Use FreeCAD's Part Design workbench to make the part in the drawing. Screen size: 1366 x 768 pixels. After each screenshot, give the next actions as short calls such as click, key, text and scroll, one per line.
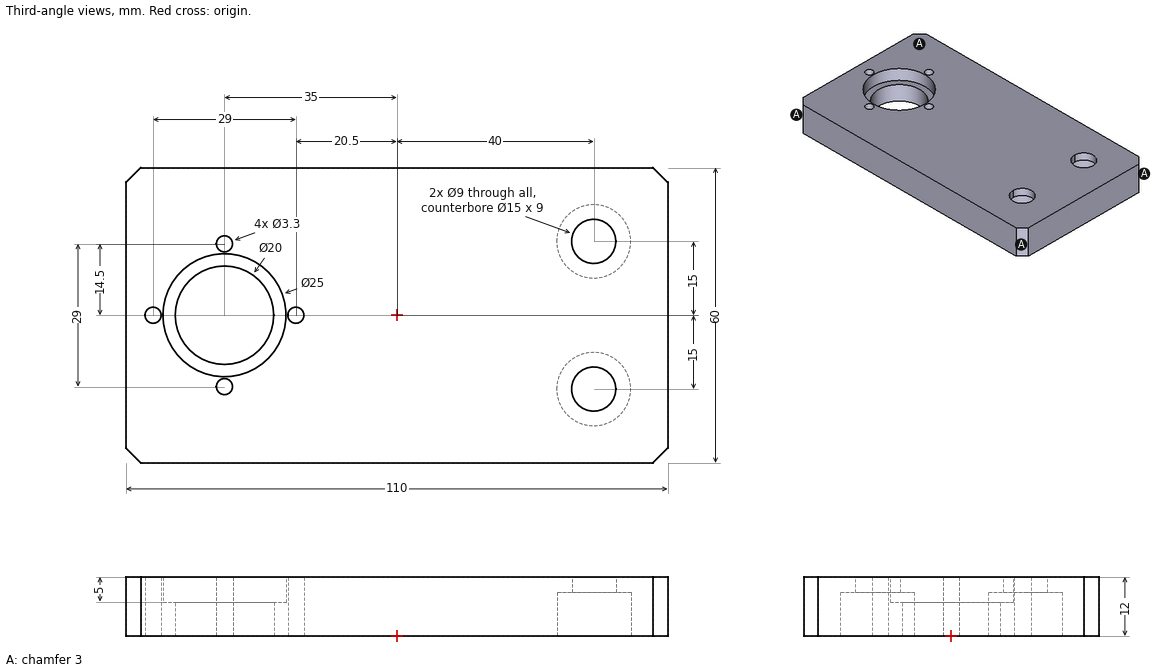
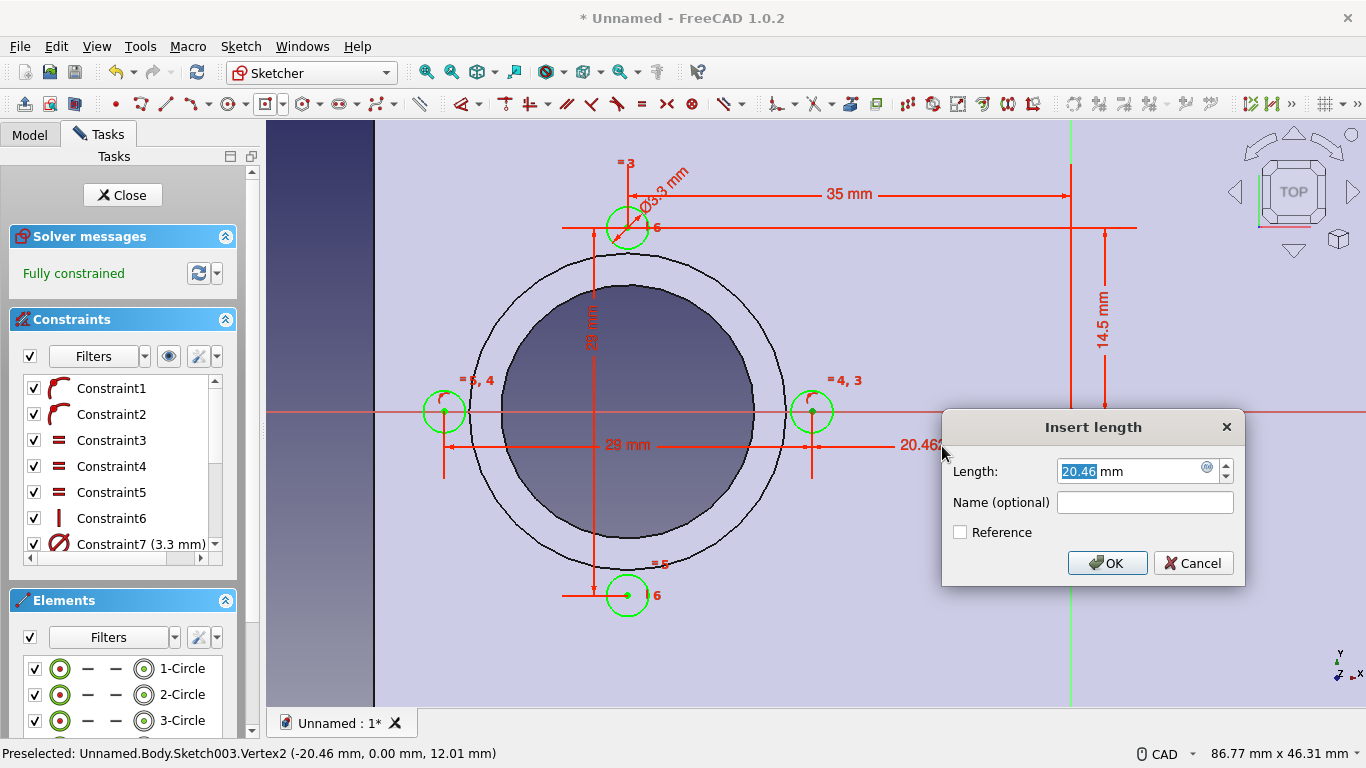
text(20.5)
key(Return)
key(Escape)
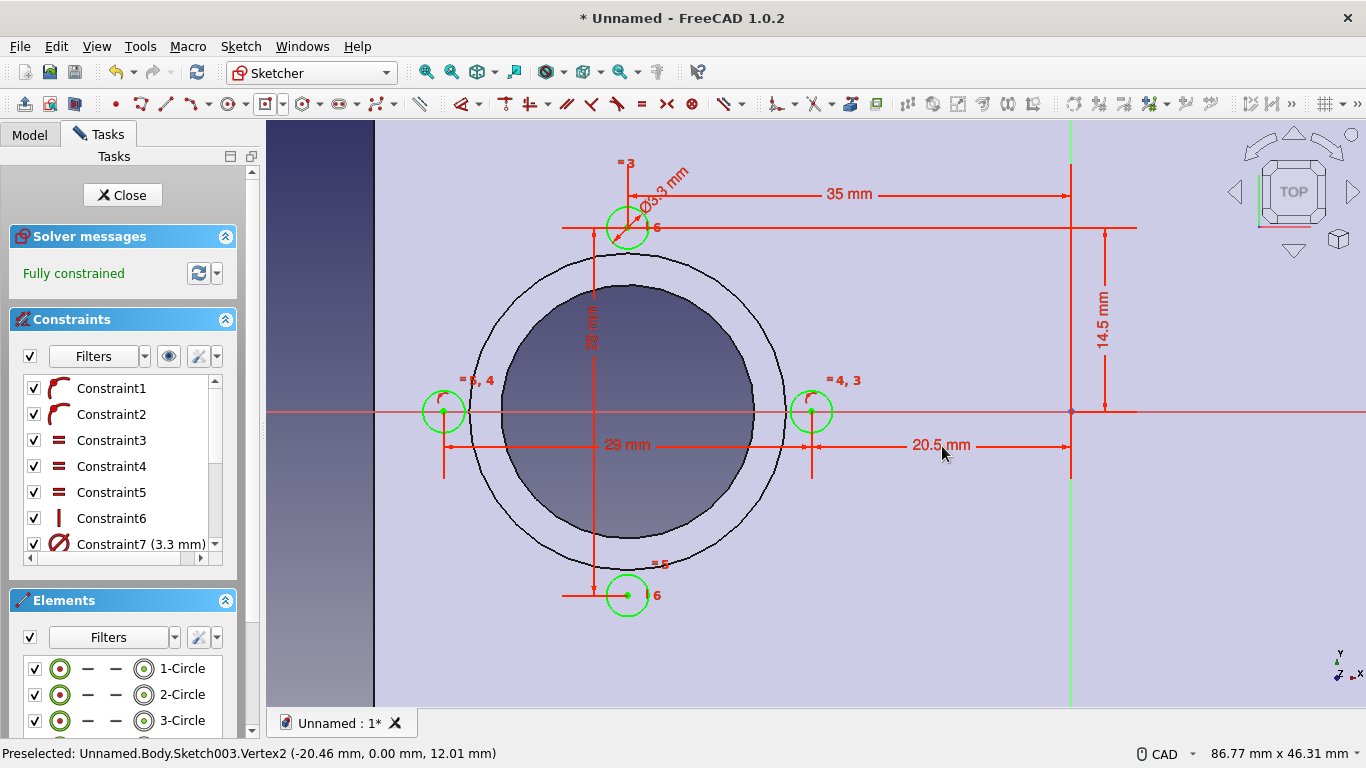
click(123, 195)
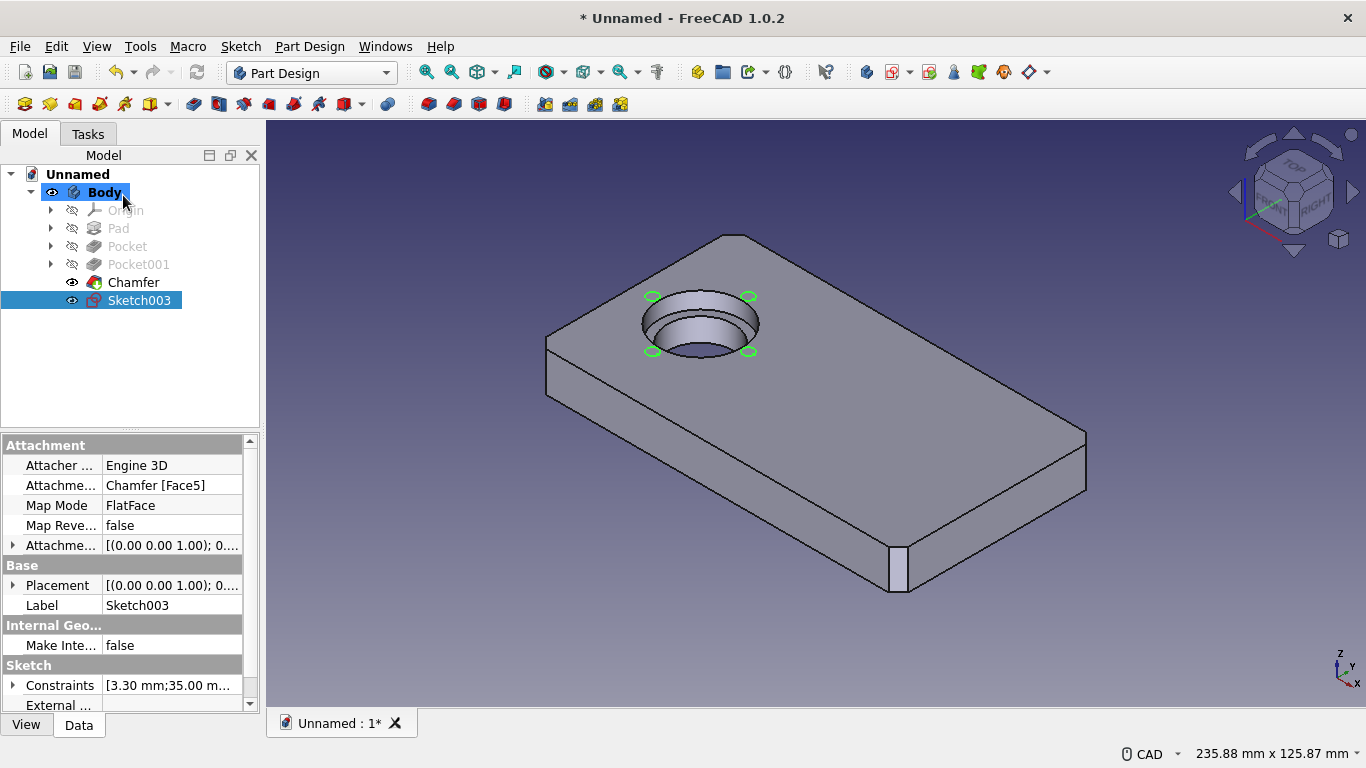
click(194, 104)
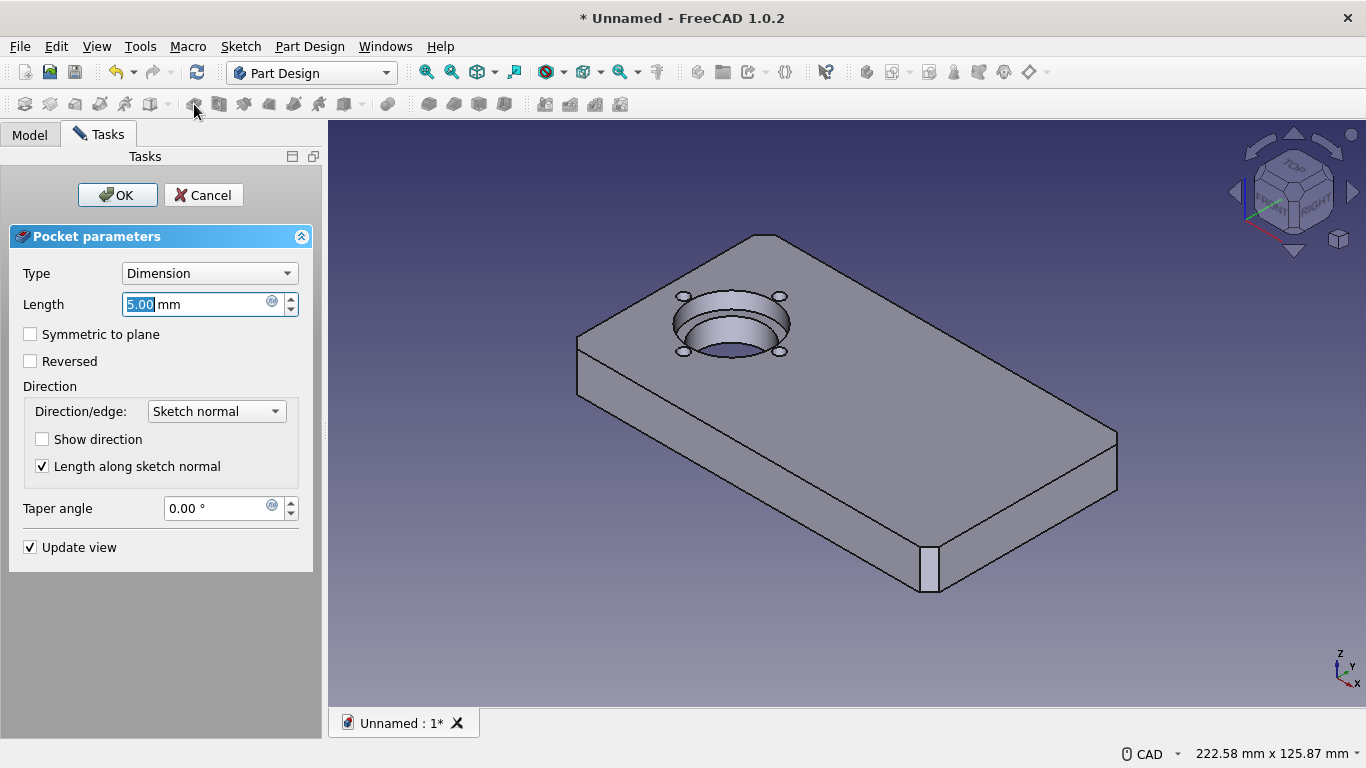
click(210, 274)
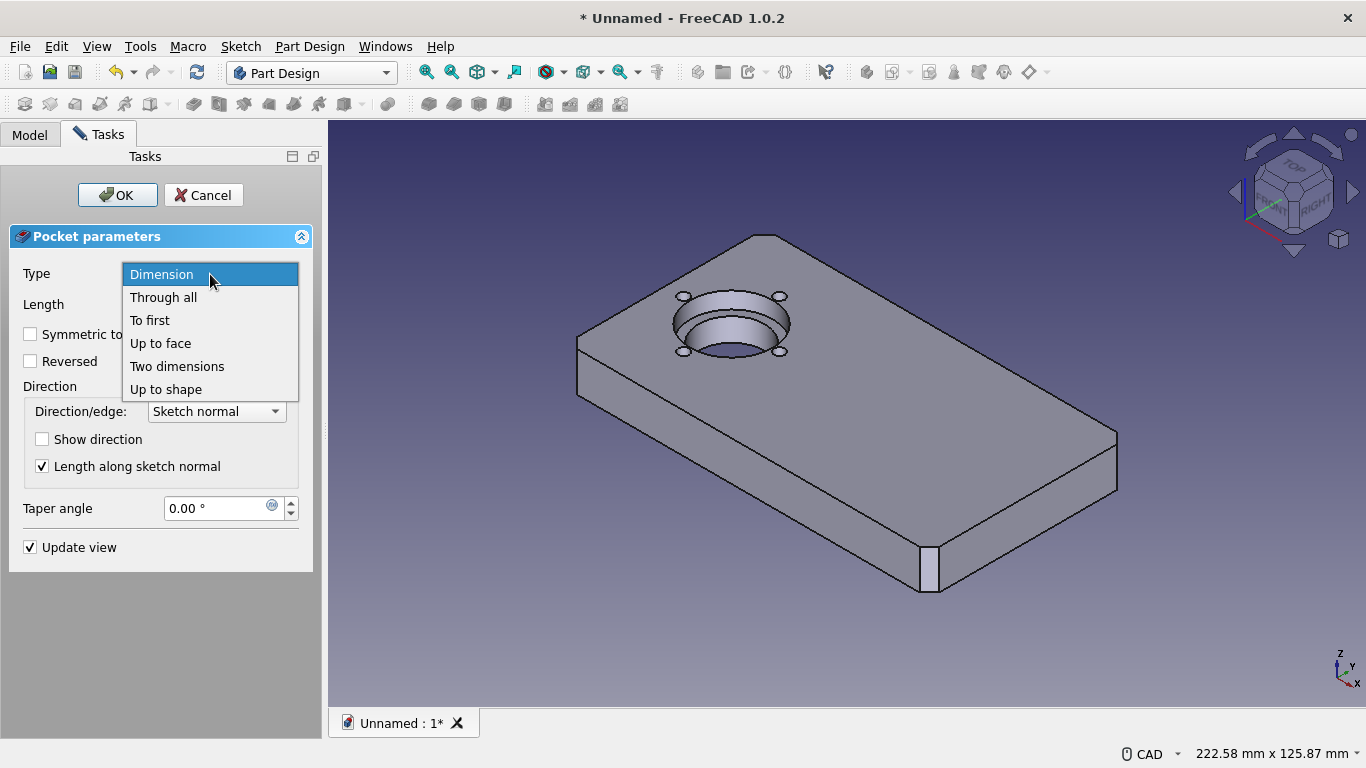
click(208, 298)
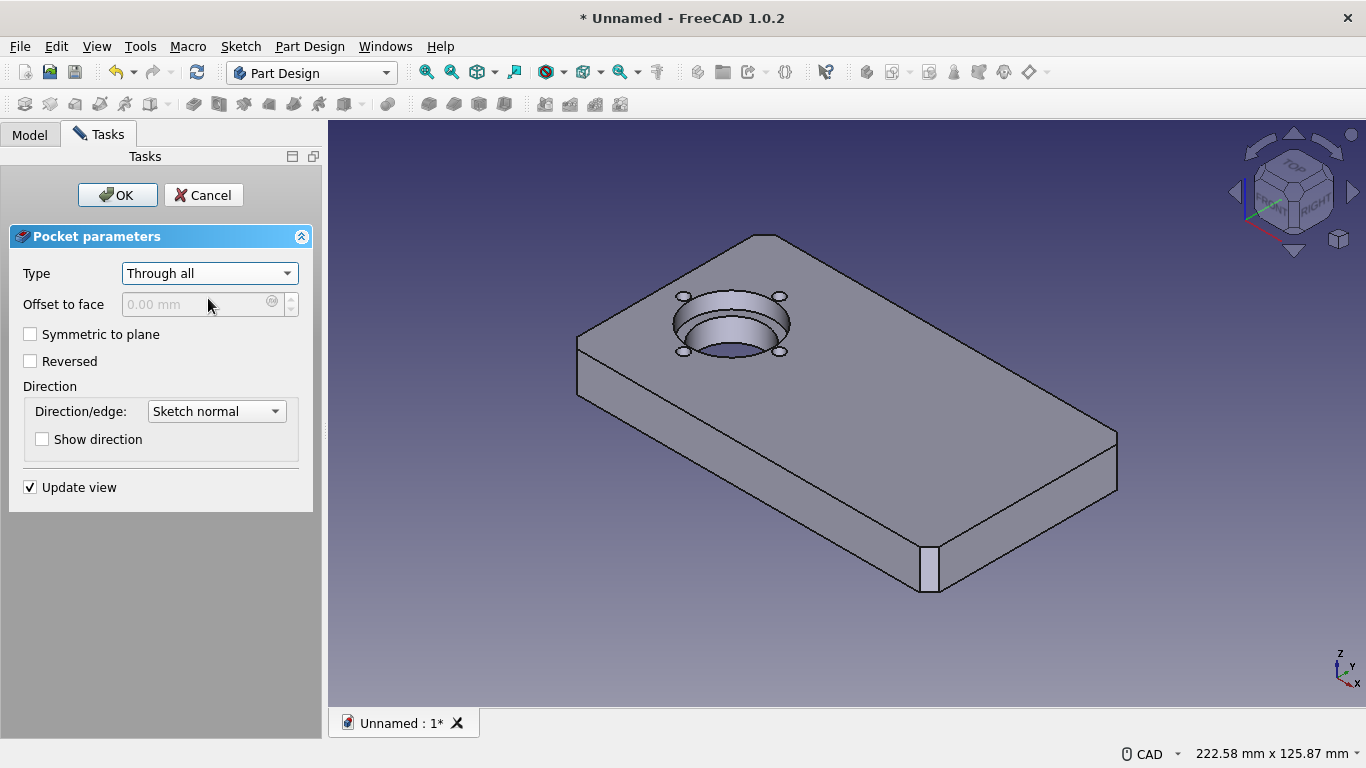
click(118, 195)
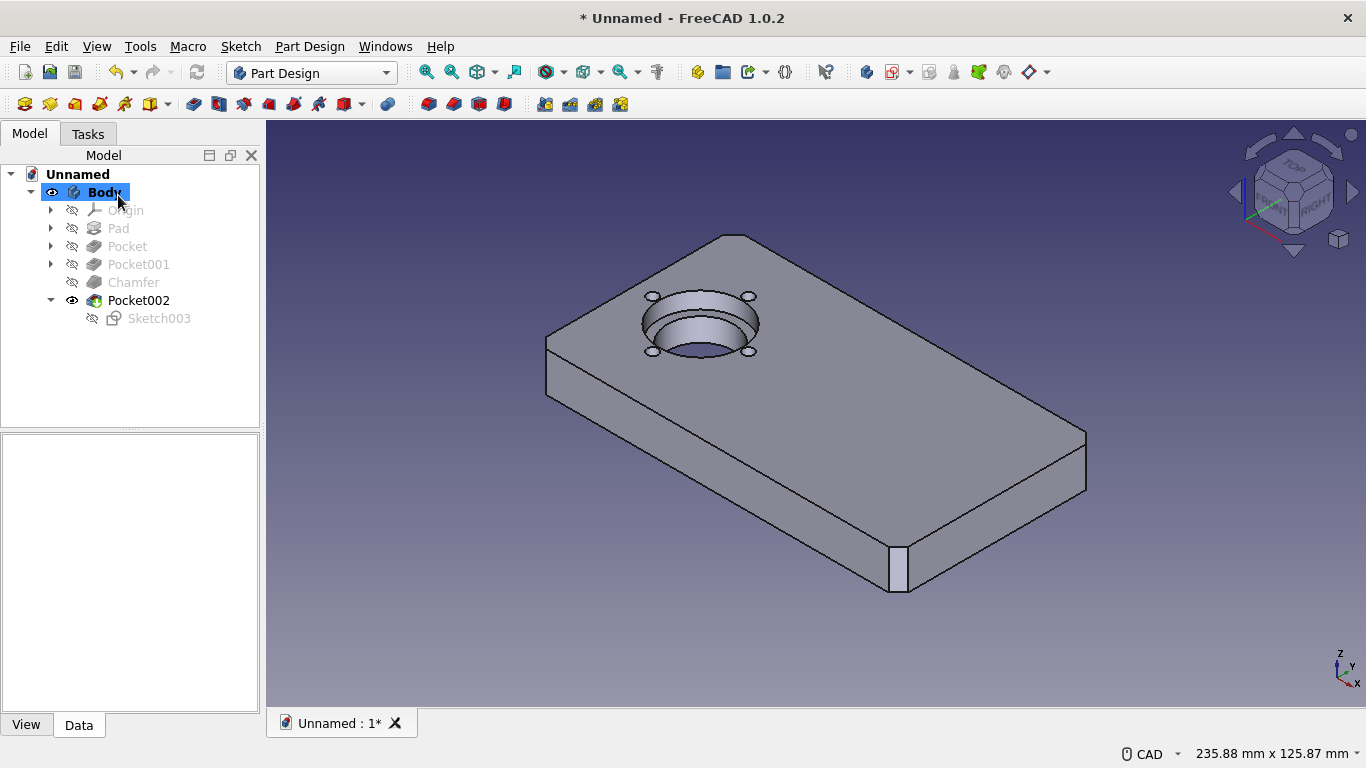
click(892, 72)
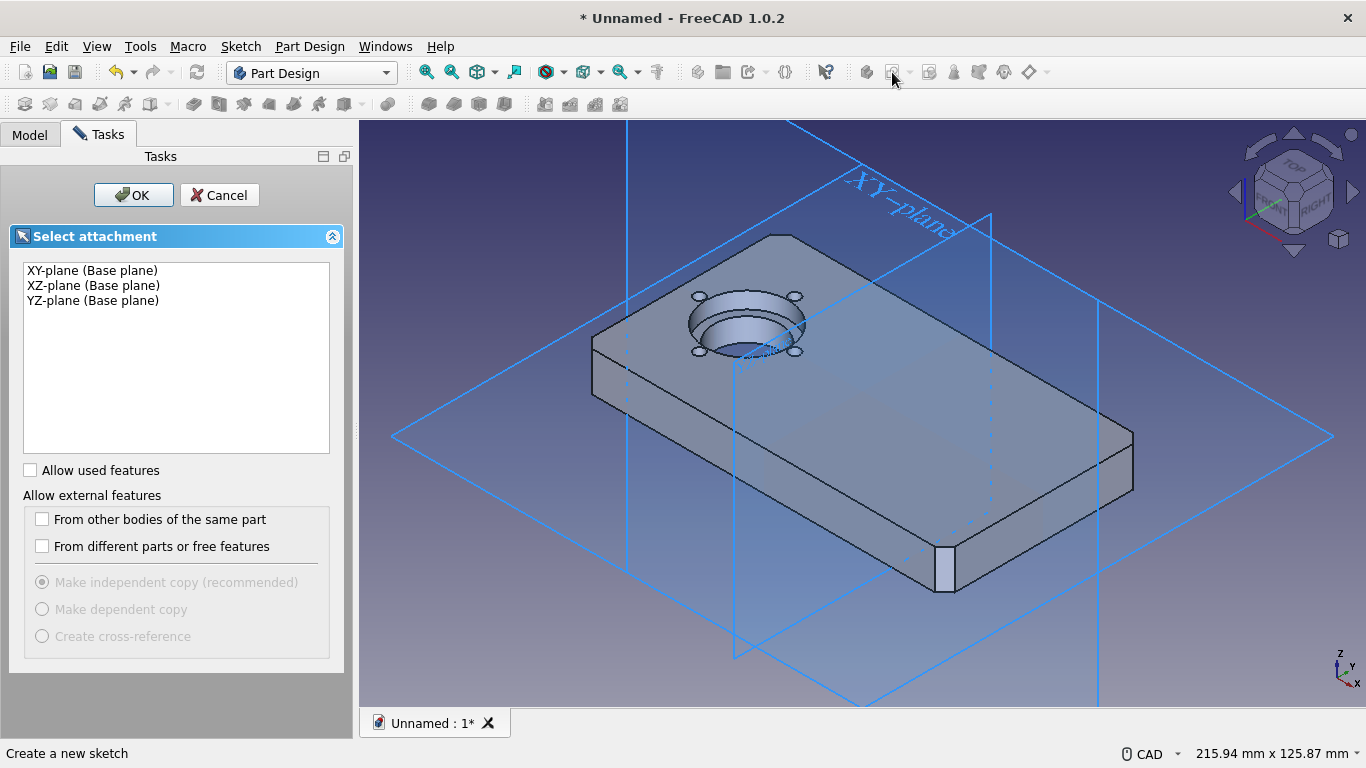
click(84, 270)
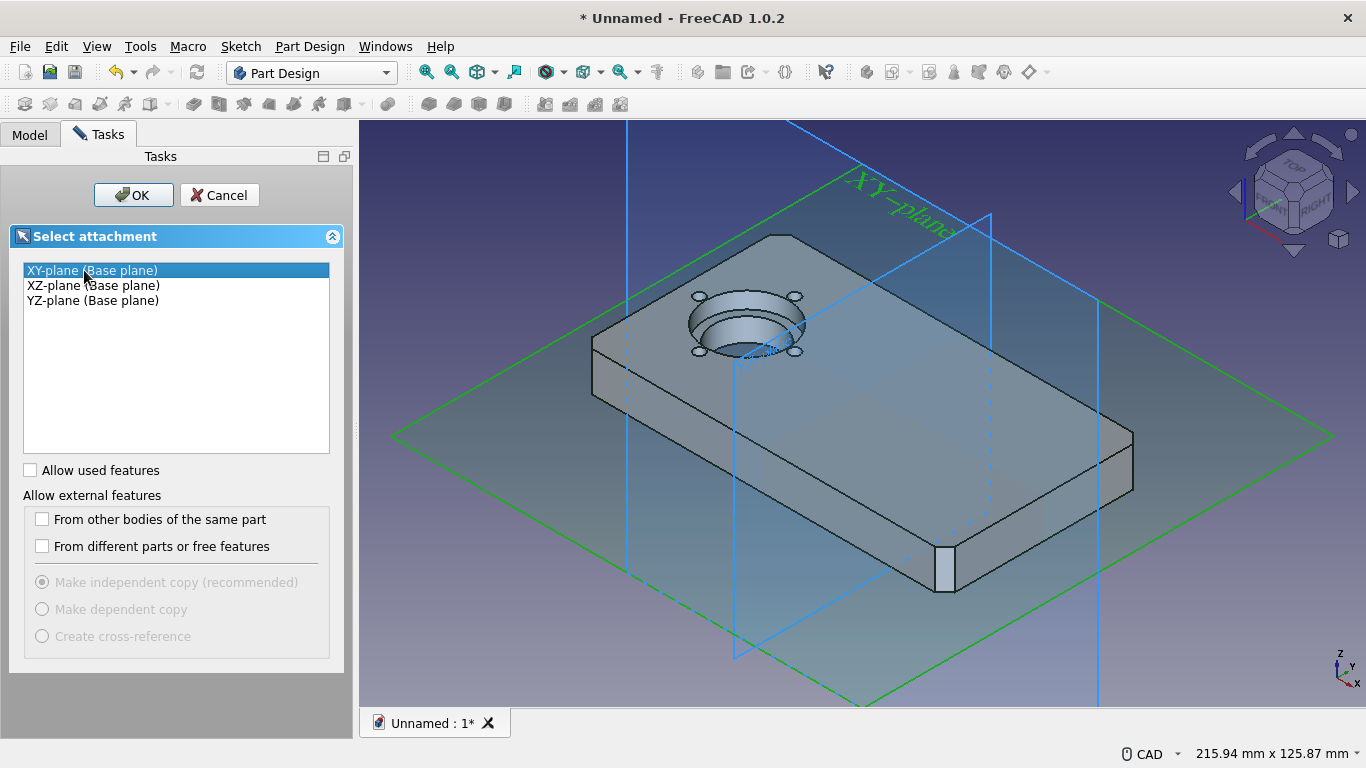
click(134, 195)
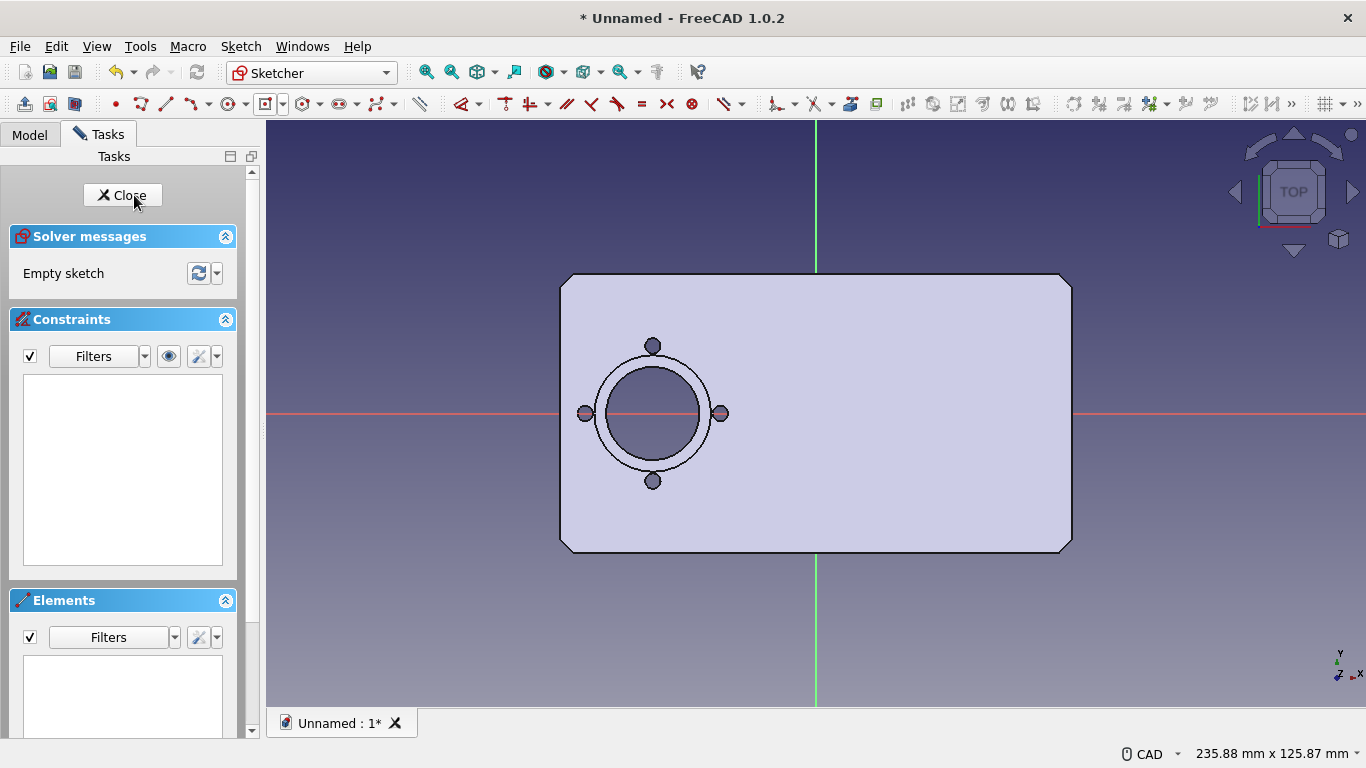
click(75, 104)